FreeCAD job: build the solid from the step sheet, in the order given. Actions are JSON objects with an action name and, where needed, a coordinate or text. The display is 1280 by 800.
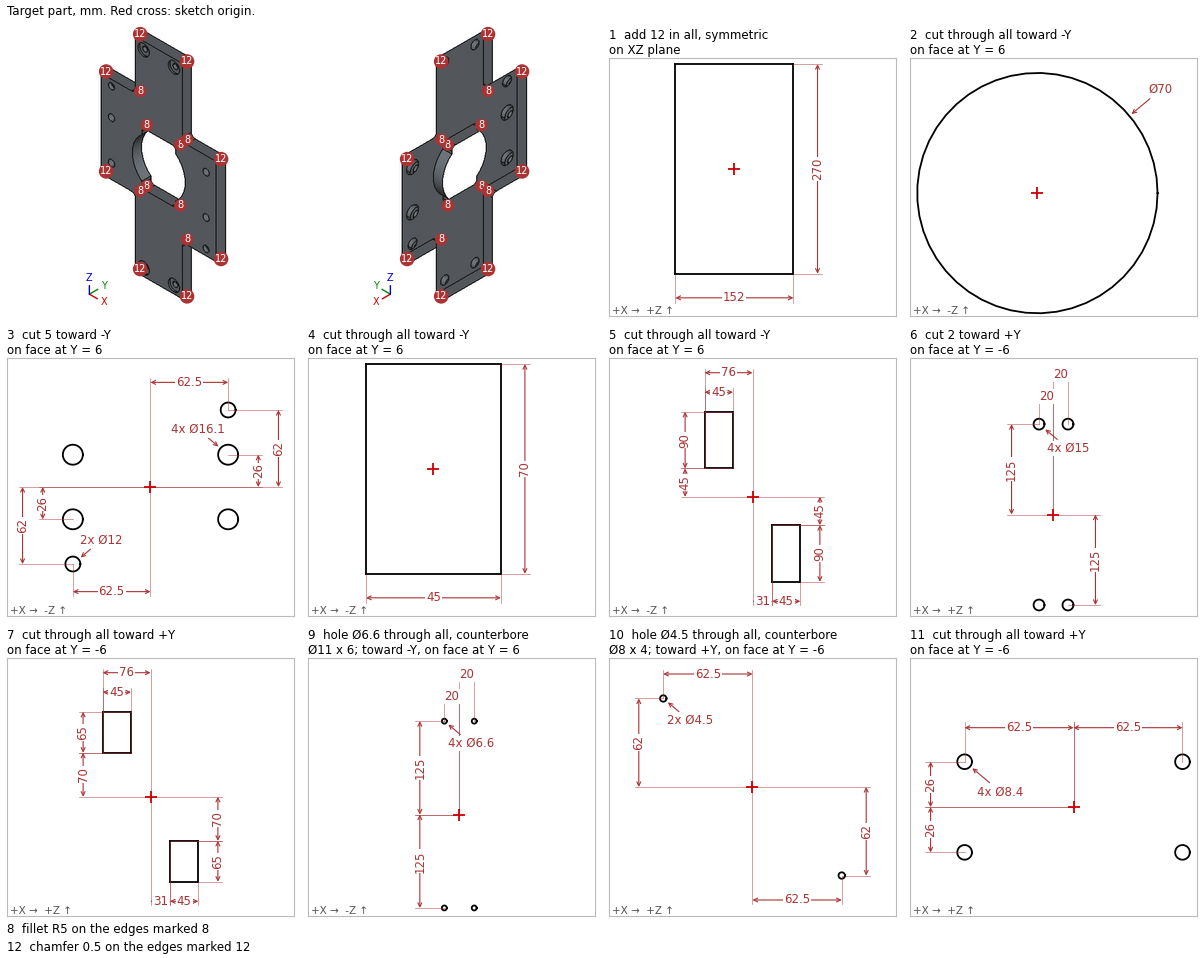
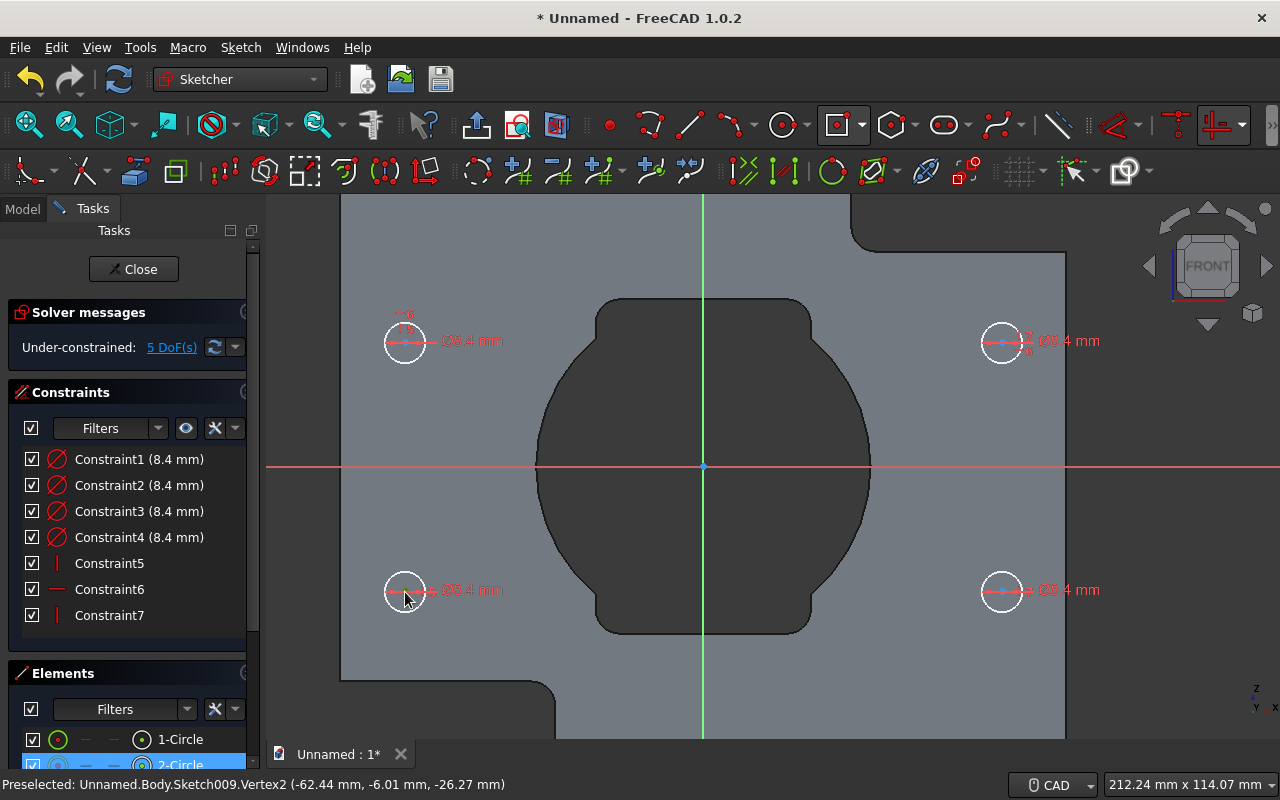
{"action": "left_click", "coordinate": [1002, 592]}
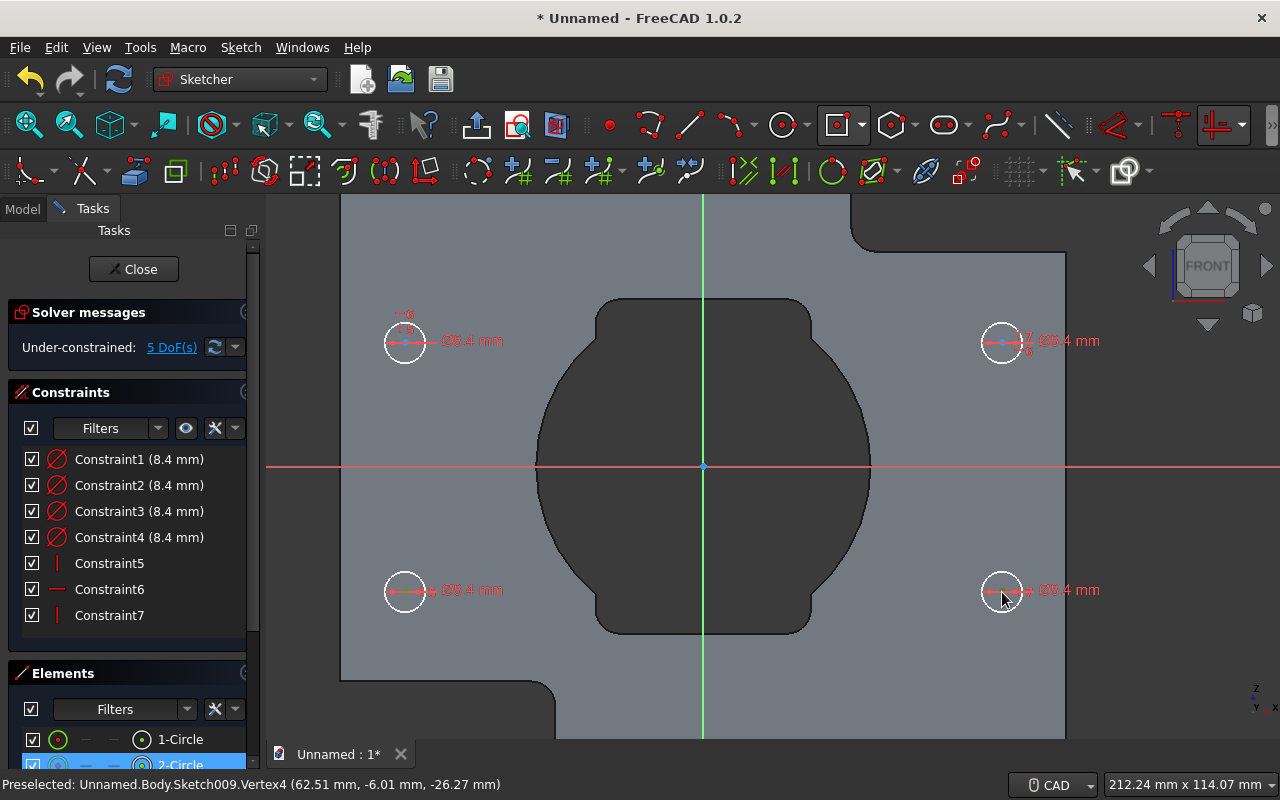
{"action": "key", "text": "h"}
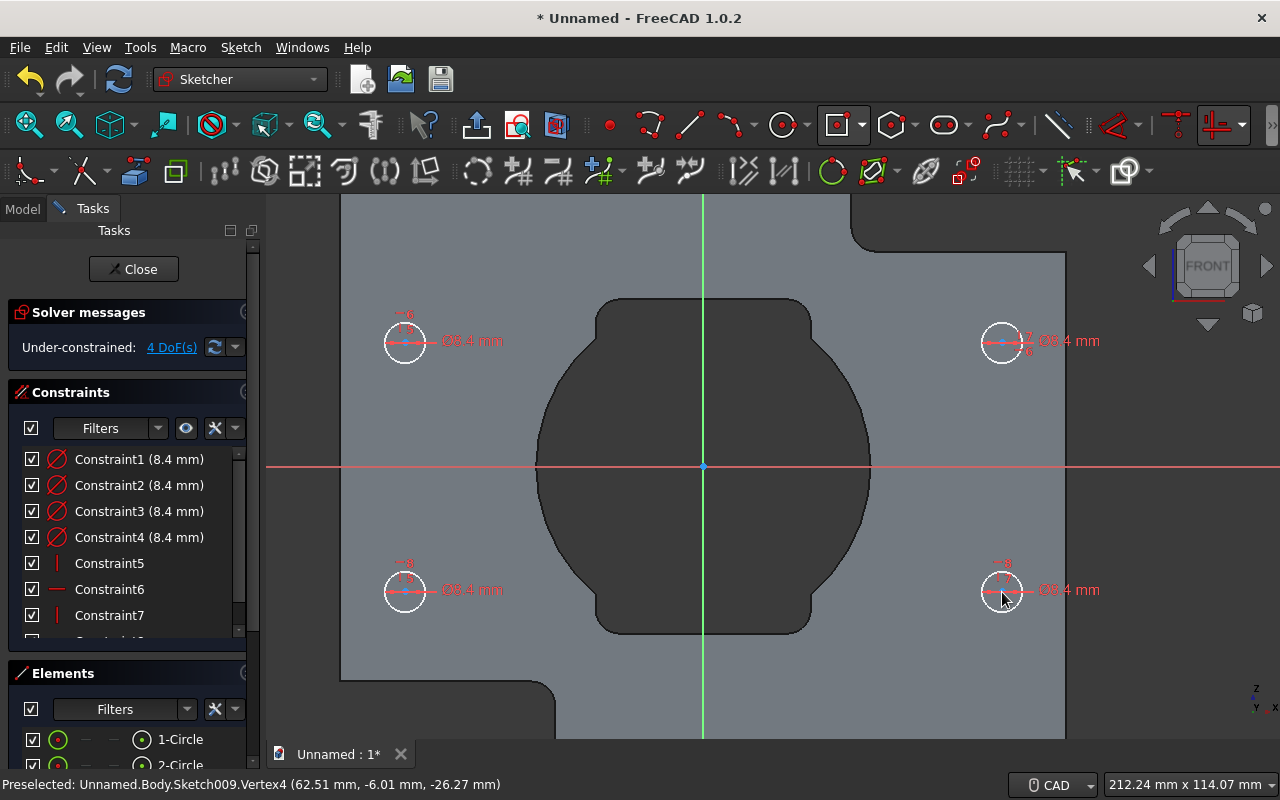
{"action": "key", "text": "d"}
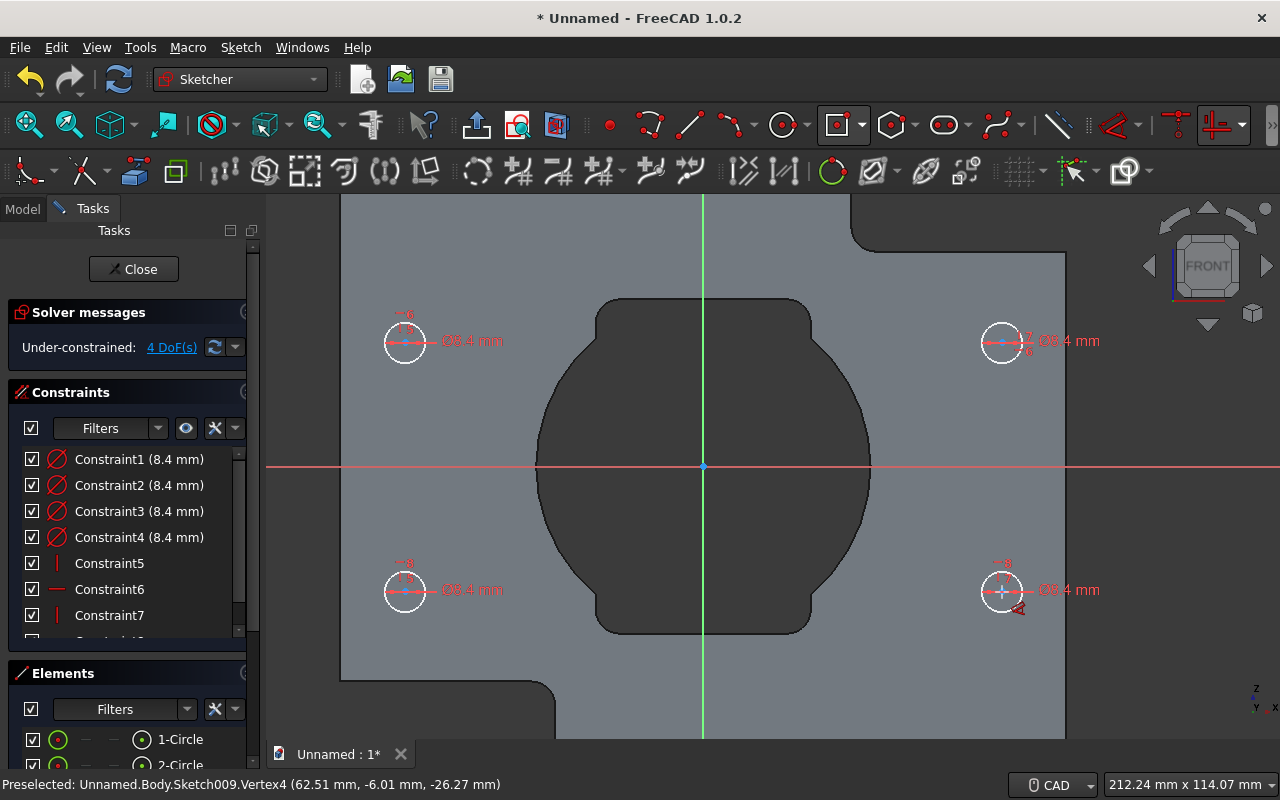
{"action": "left_click", "coordinate": [405, 343]}
{"action": "left_click", "coordinate": [371, 405]}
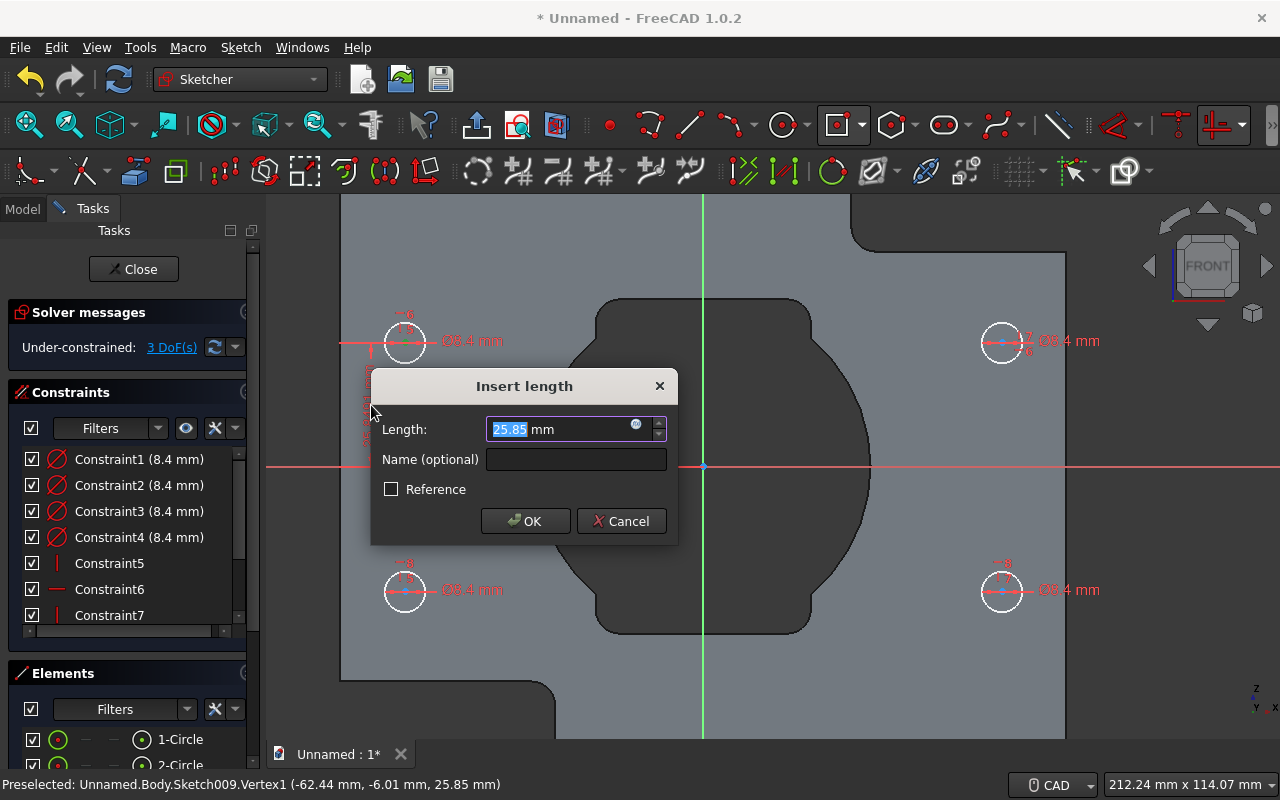
{"action": "type", "text": "26"}
{"action": "key", "text": "Return"}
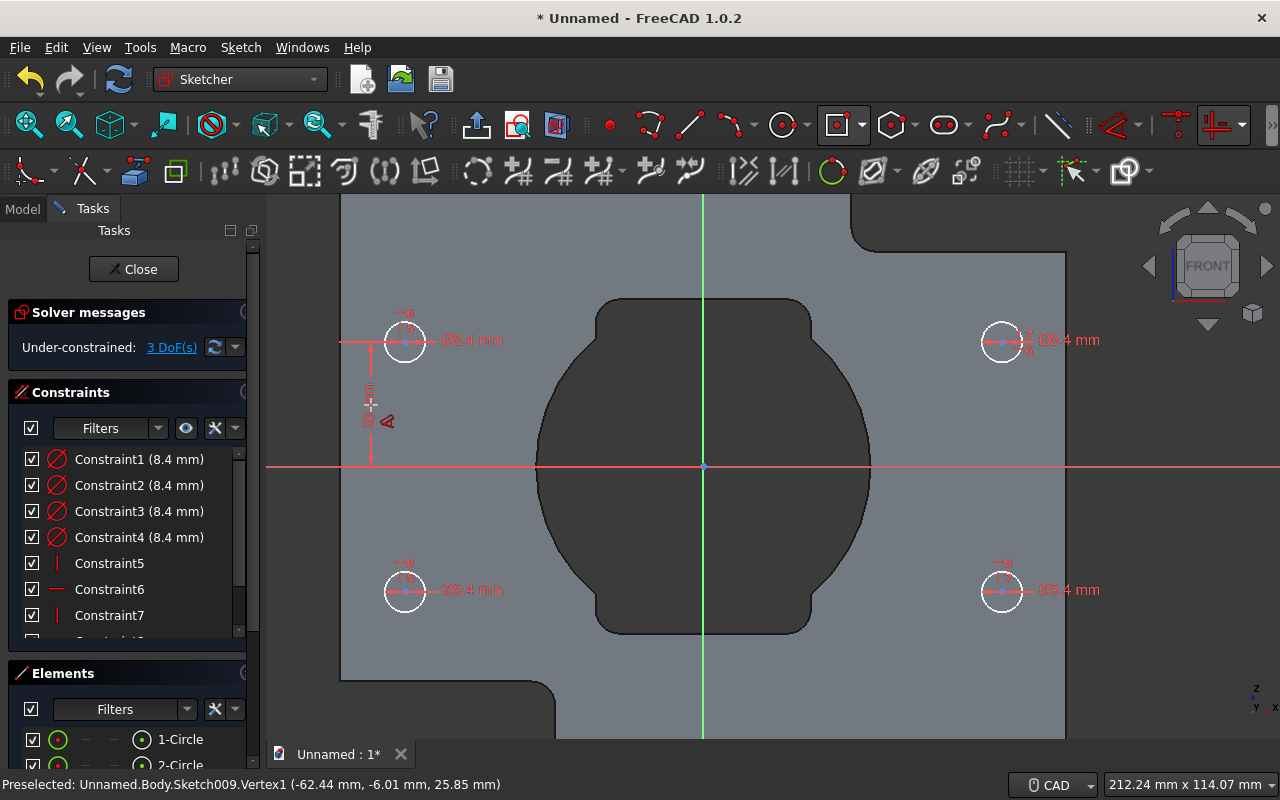
{"action": "left_click", "coordinate": [405, 592]}
{"action": "left_click", "coordinate": [371, 529]}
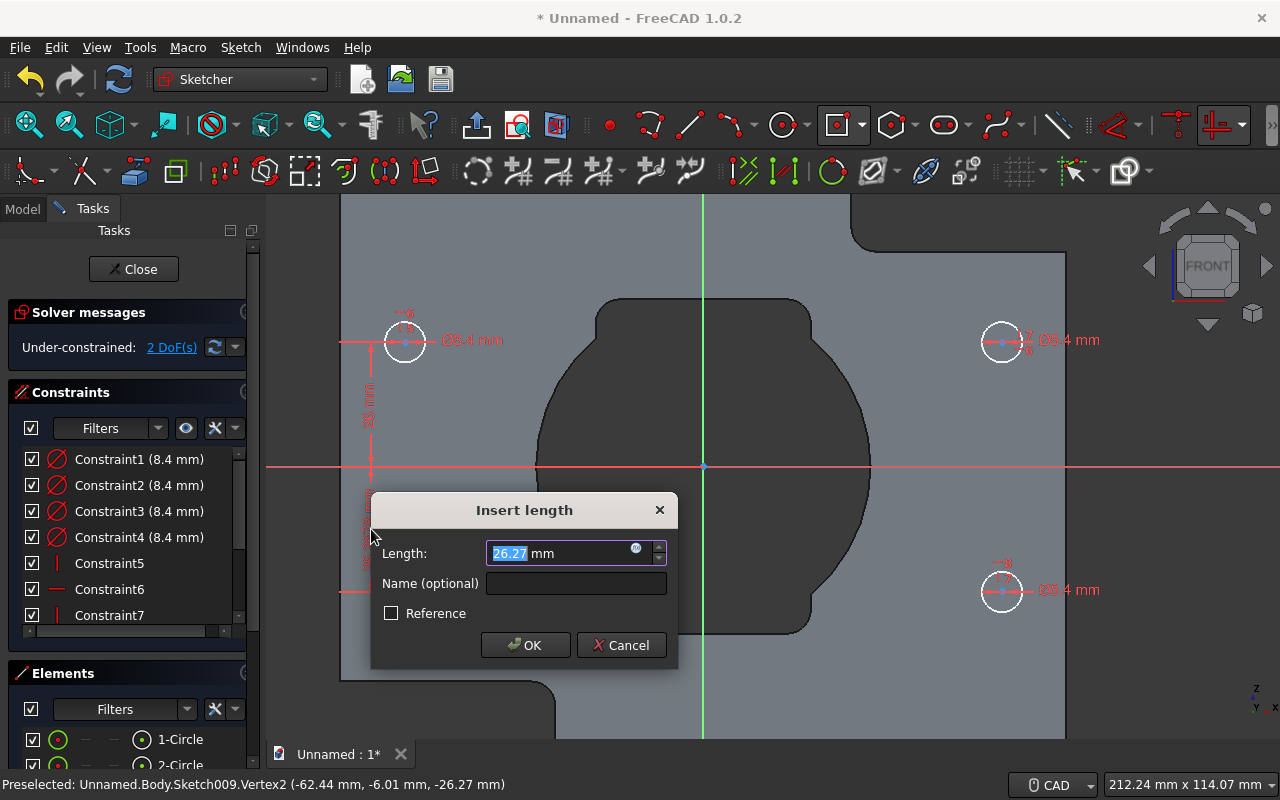
{"action": "type", "text": "26"}
{"action": "key", "text": "Return"}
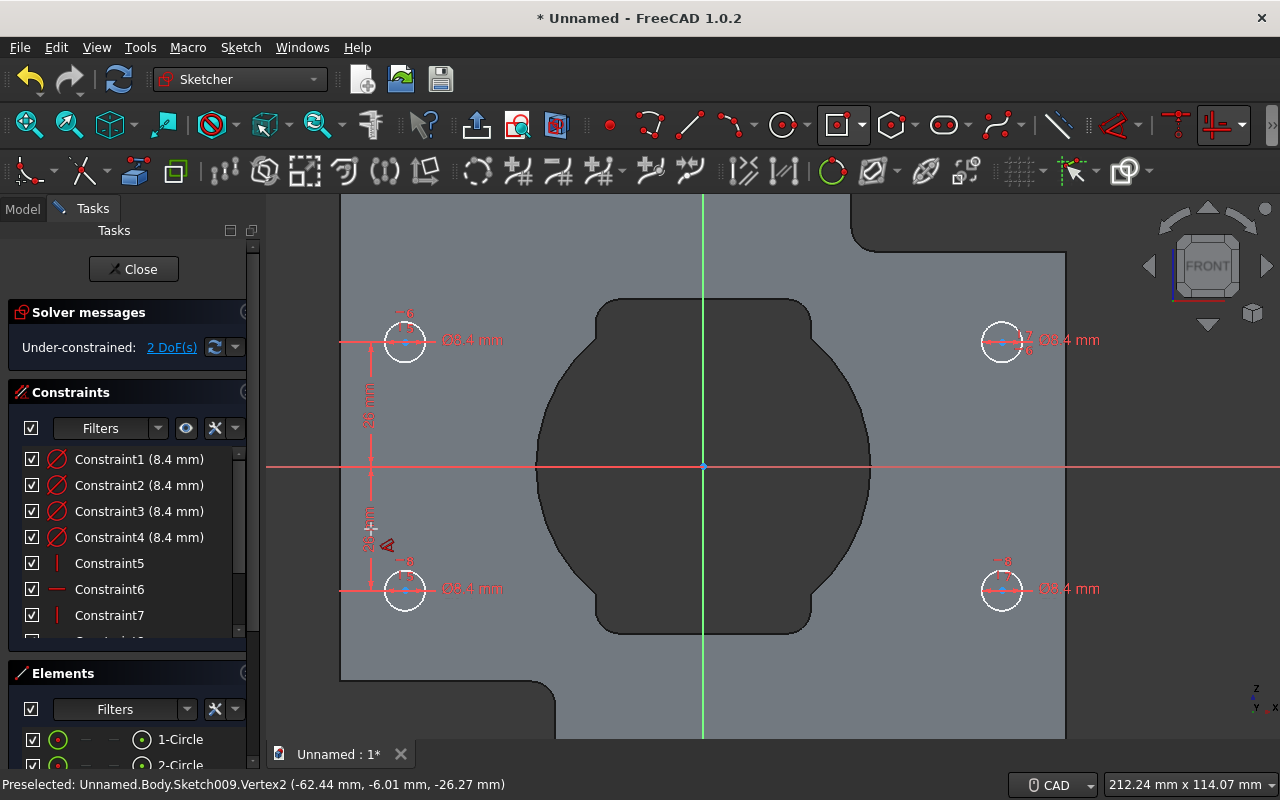
{"action": "left_click", "coordinate": [405, 342]}
{"action": "left_click", "coordinate": [554, 308]}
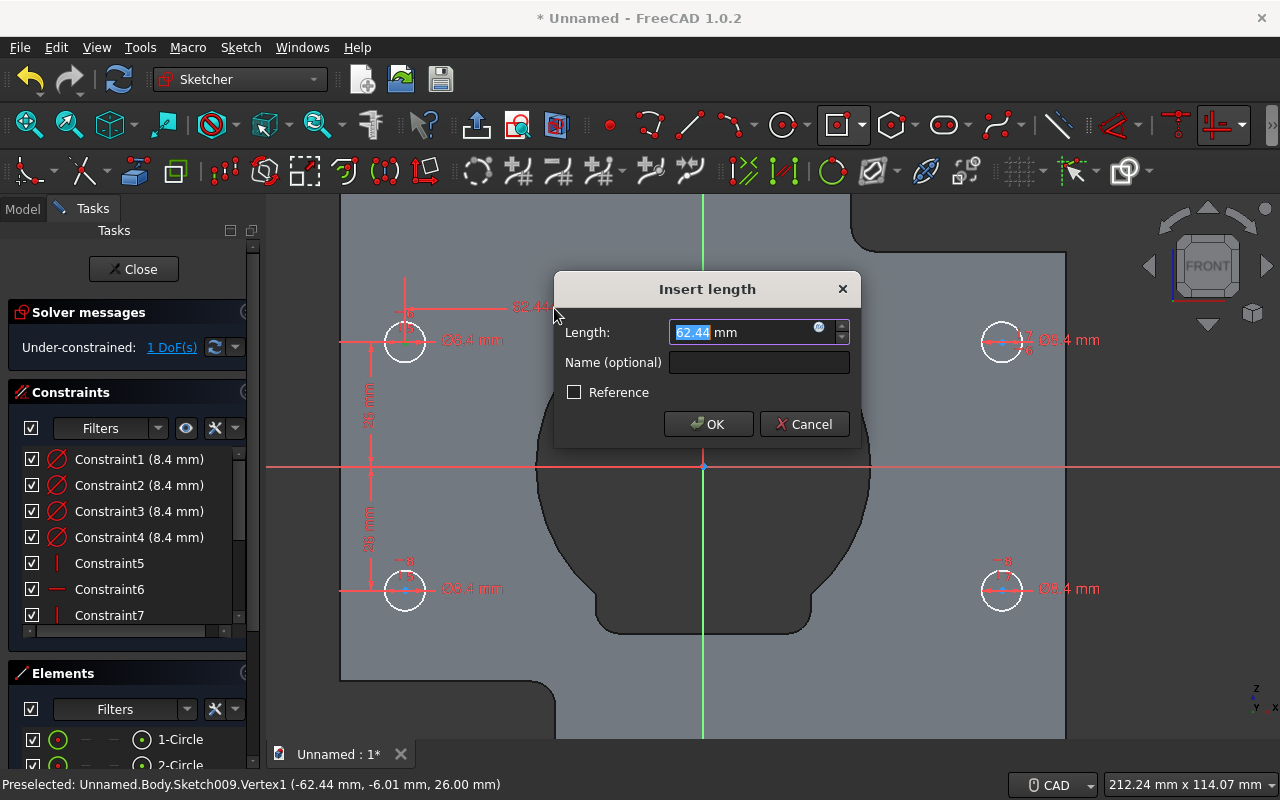
{"action": "type", "text": "62.5"}
{"action": "key", "text": "Return"}